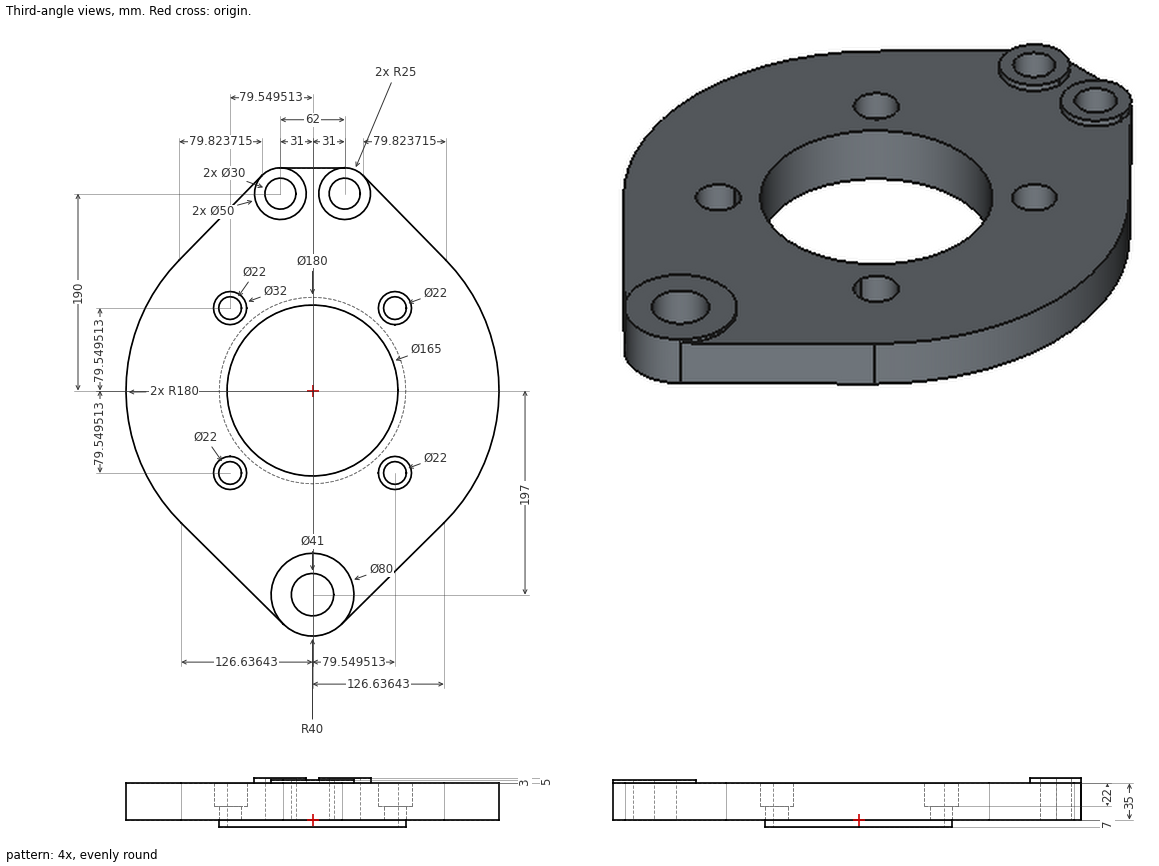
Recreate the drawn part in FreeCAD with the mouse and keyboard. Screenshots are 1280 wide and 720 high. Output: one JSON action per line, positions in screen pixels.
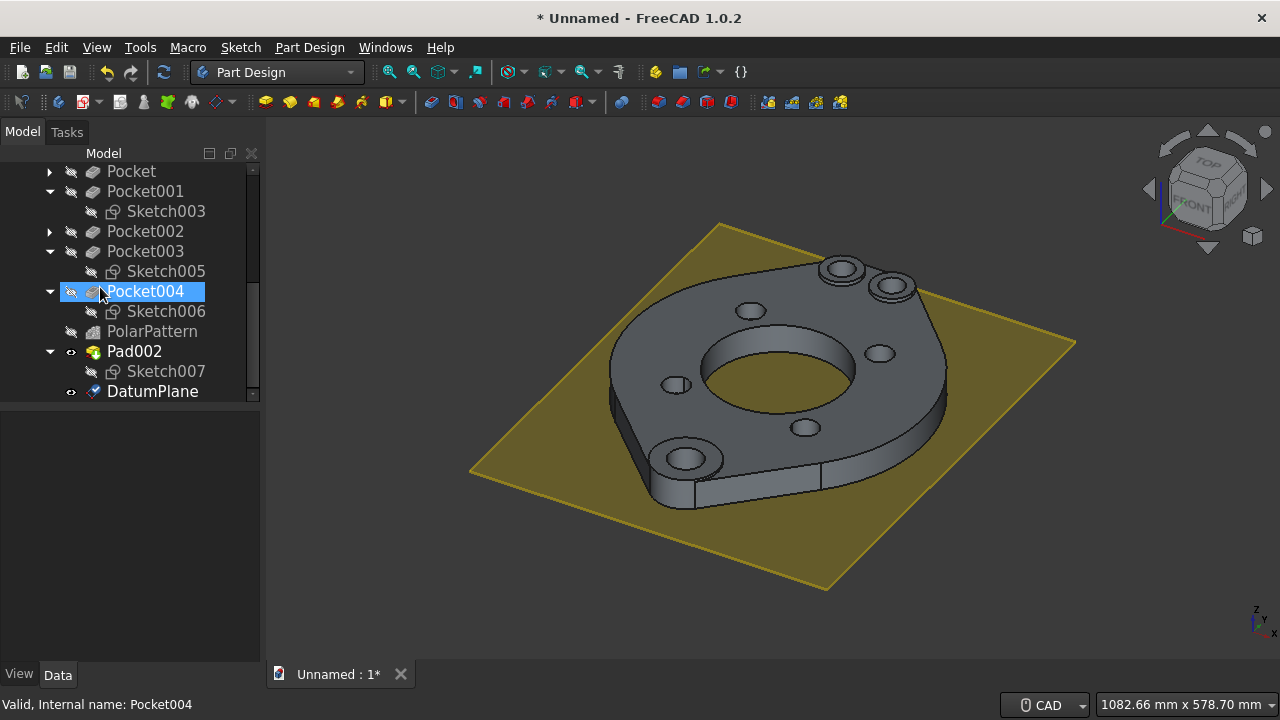
{"action": "left_click", "coordinate": [116, 392]}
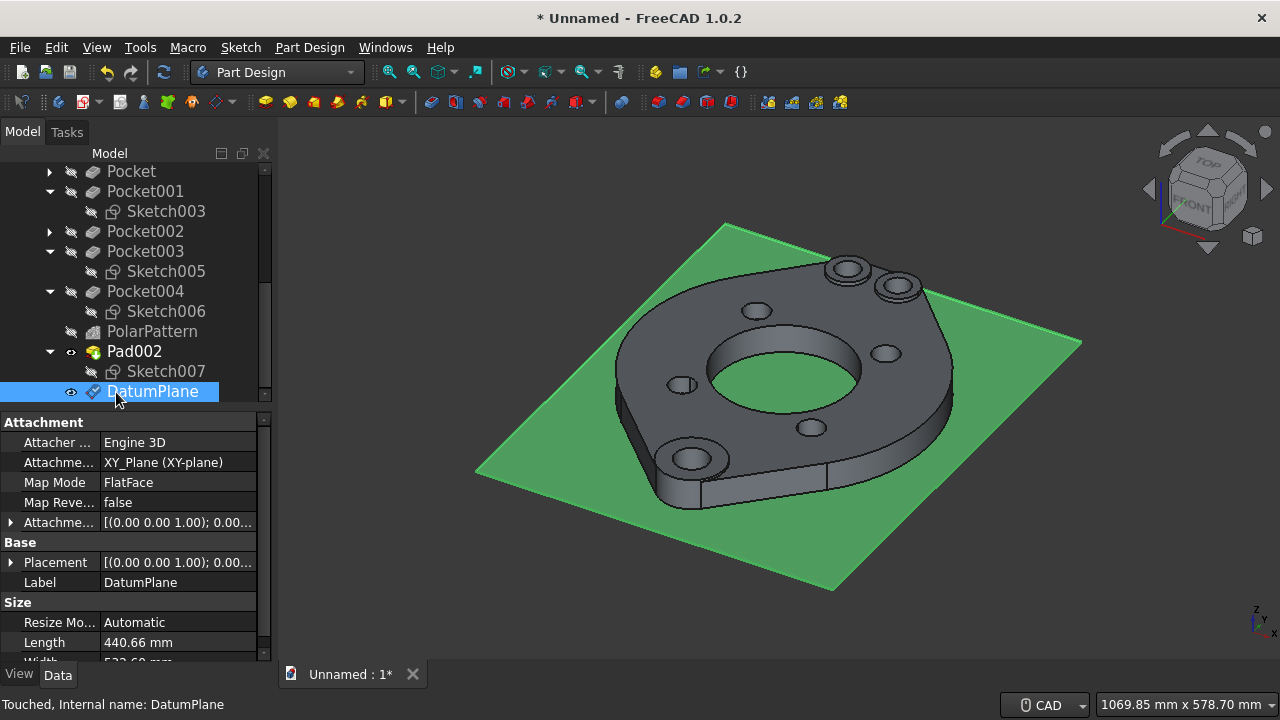
{"action": "left_click", "coordinate": [84, 102]}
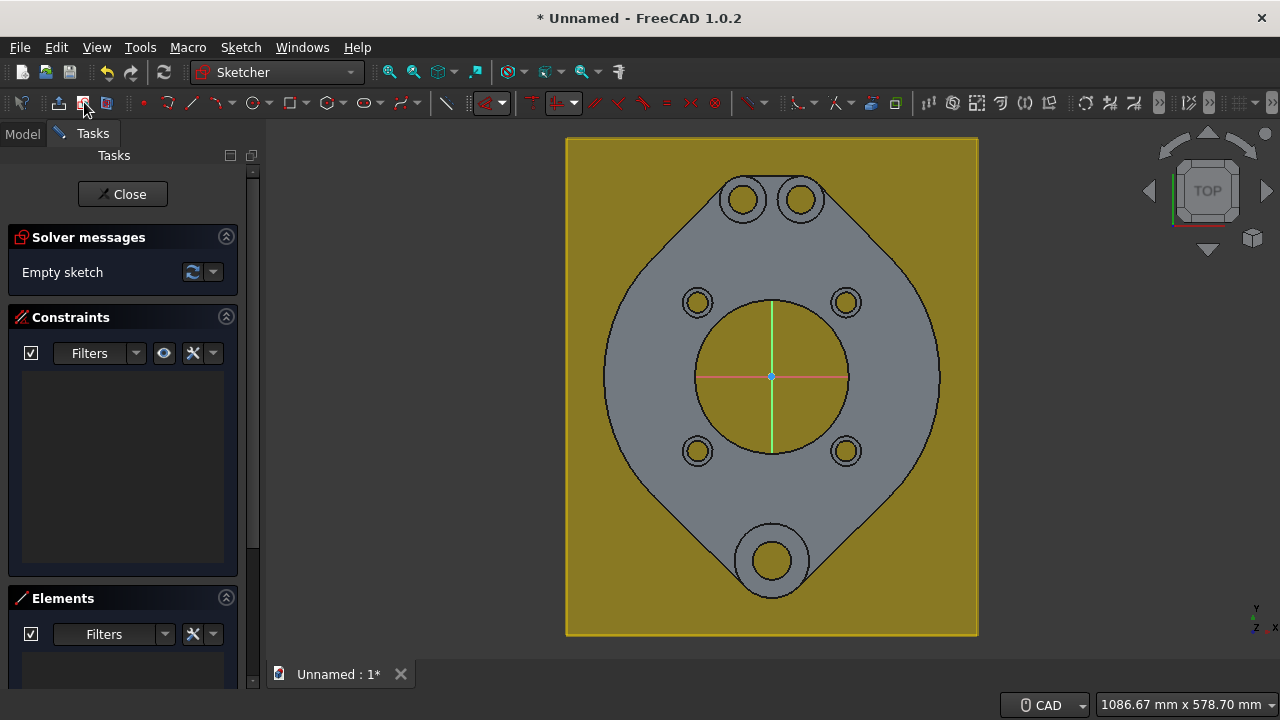
{"action": "left_click", "coordinate": [108, 104]}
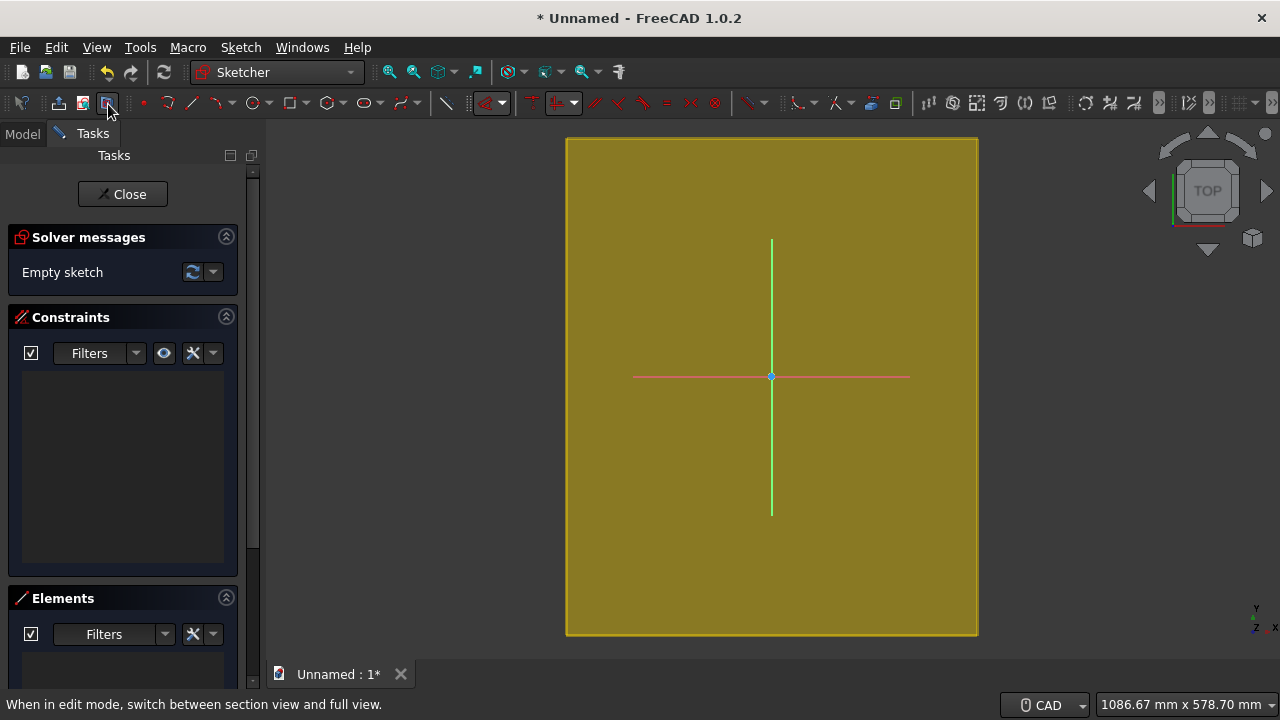
{"action": "scroll", "coordinate": [827, 367], "scroll_direction": "up", "scroll_amount": 4}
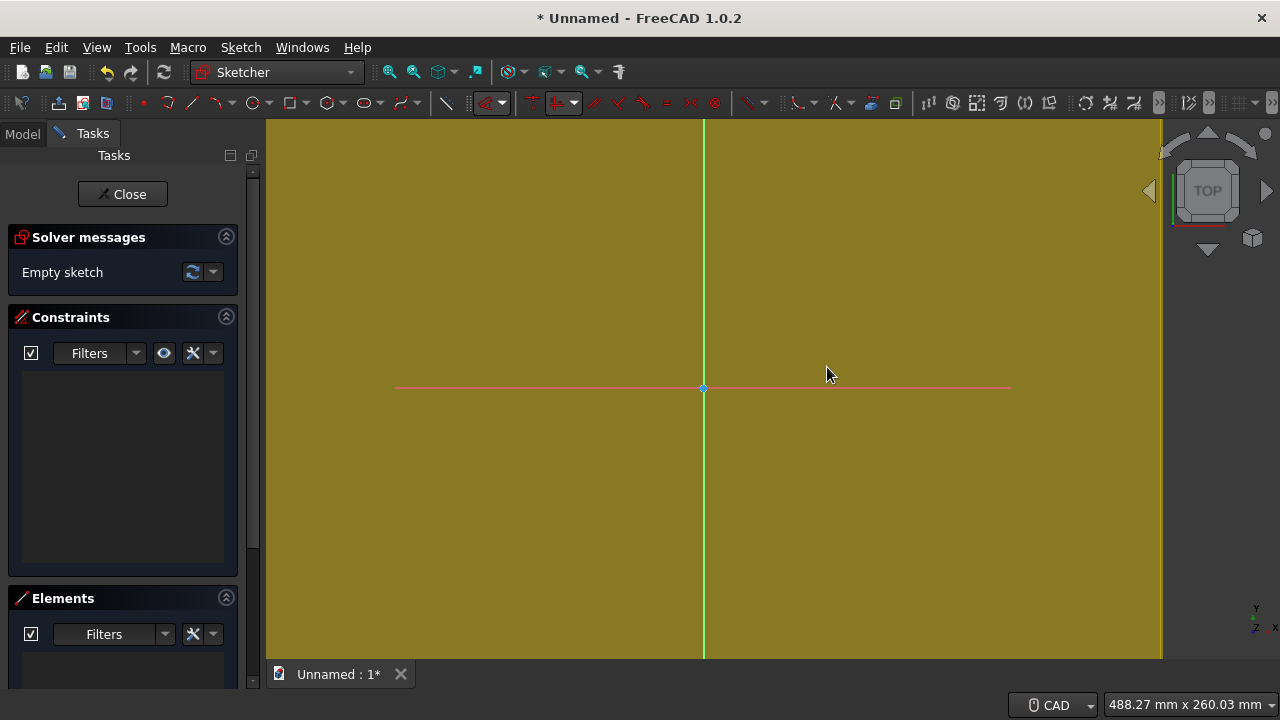
{"action": "key", "text": "g c"}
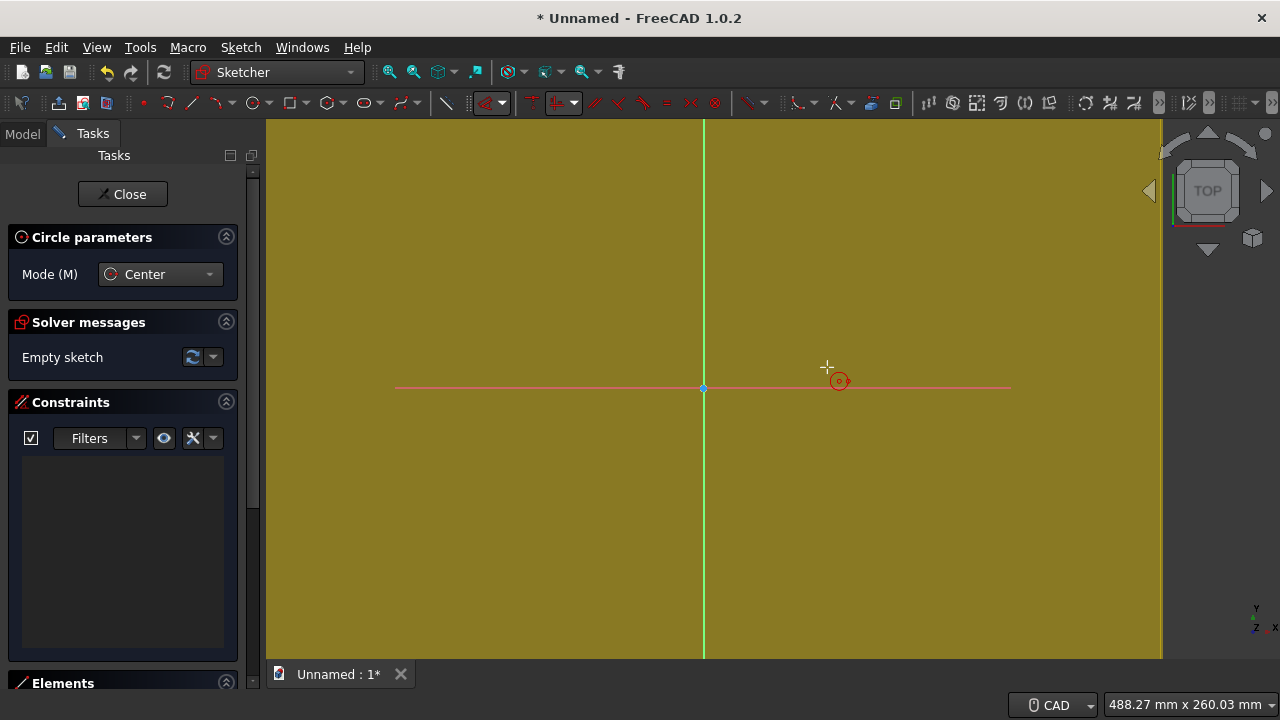
{"action": "left_click", "coordinate": [704, 388]}
{"action": "left_click", "coordinate": [836, 256]}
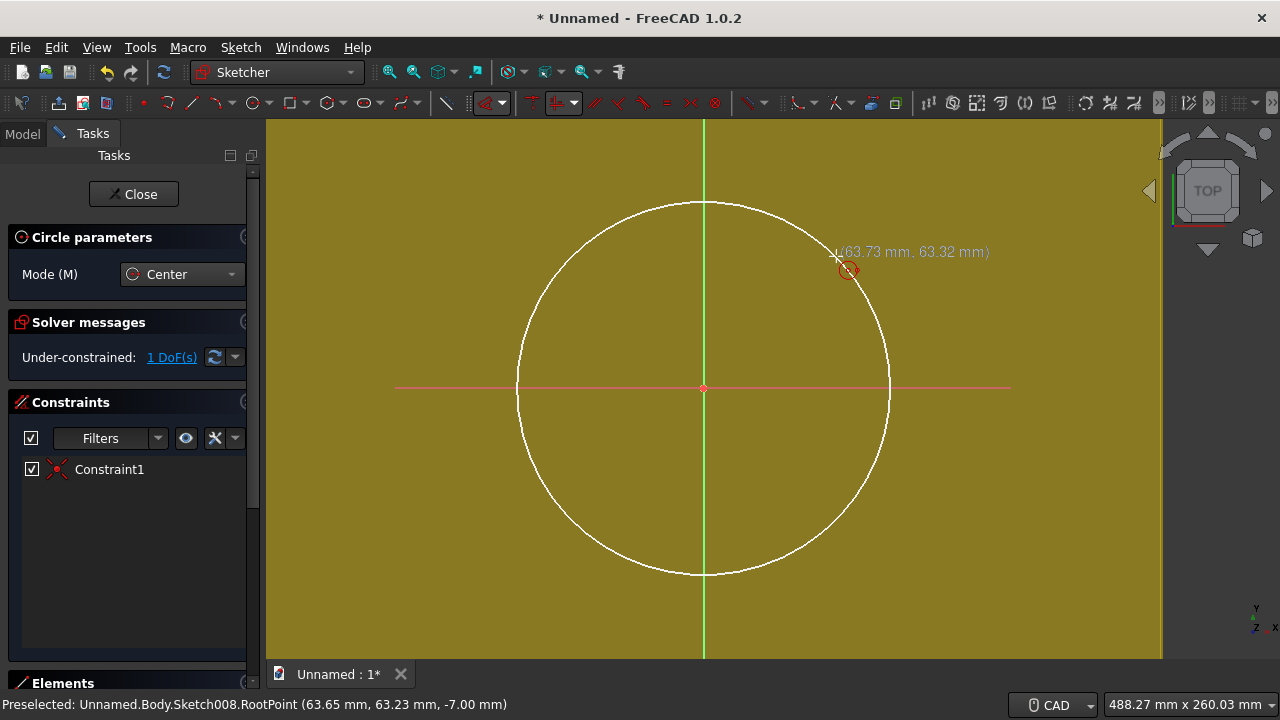
{"action": "left_click", "coordinate": [704, 388]}
{"action": "left_click", "coordinate": [825, 267]}
{"action": "key", "text": "Escape"}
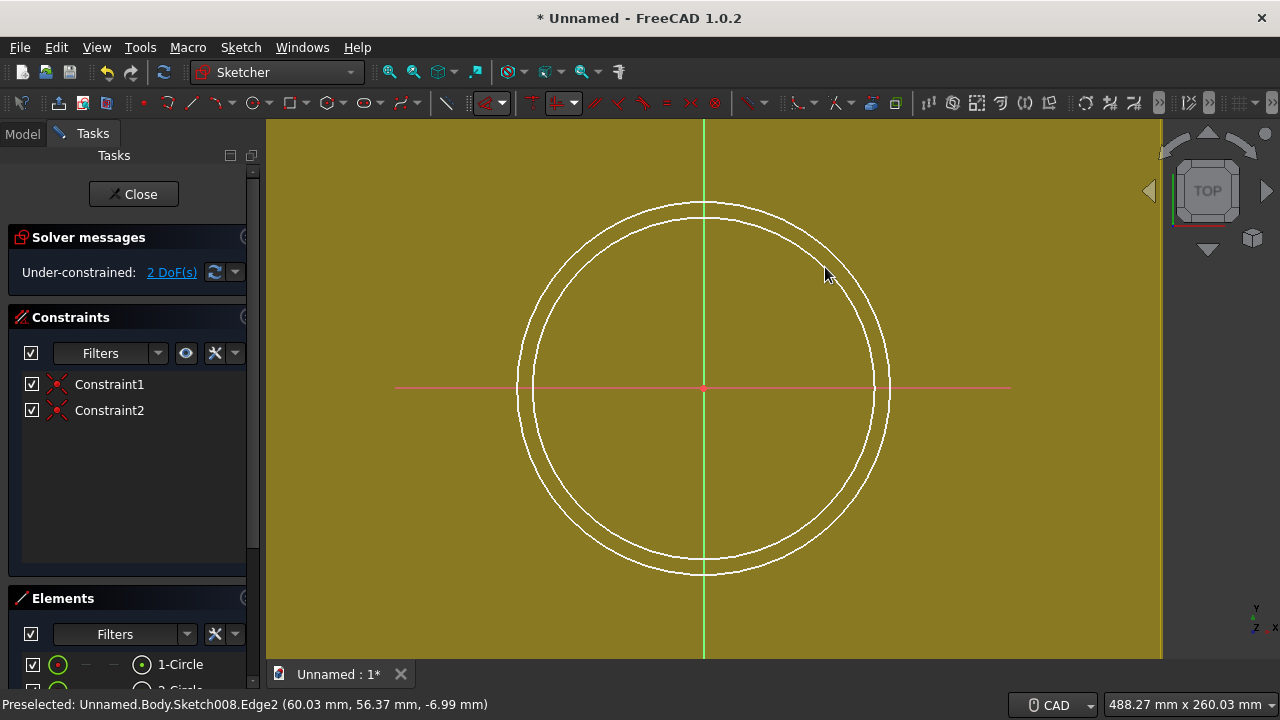
{"action": "left_click", "coordinate": [835, 256]}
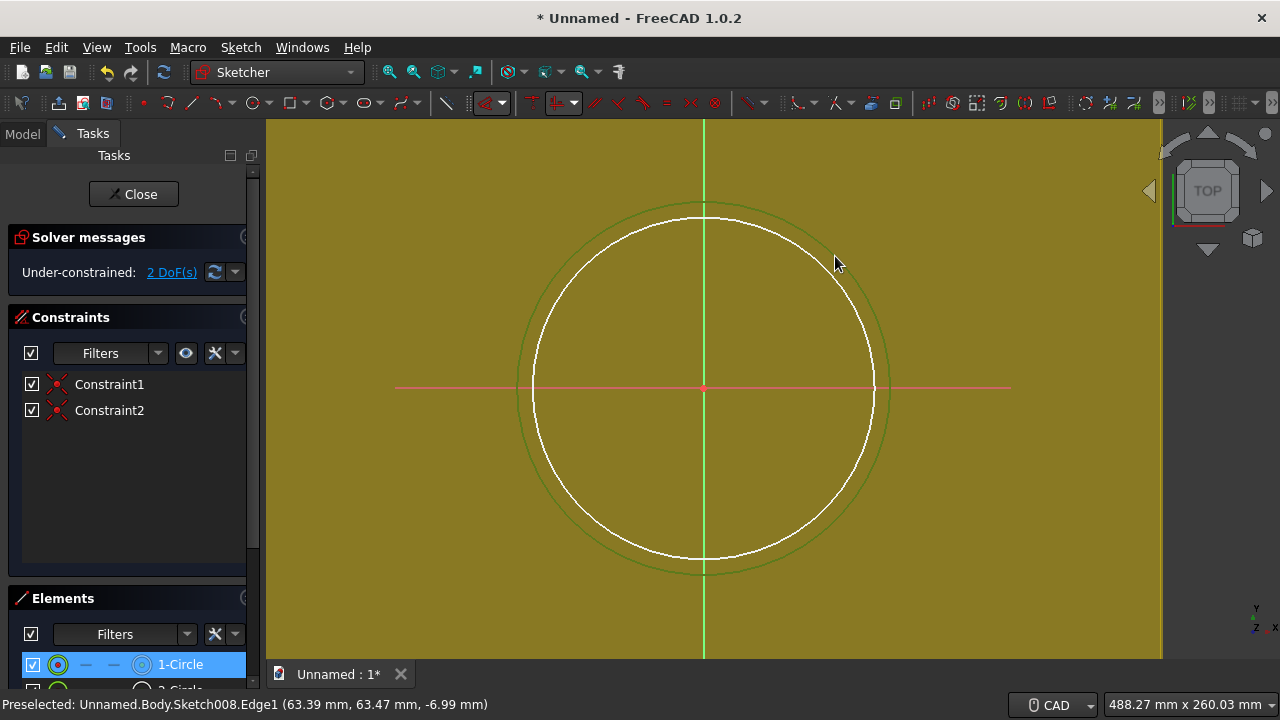
{"action": "key", "text": "k o"}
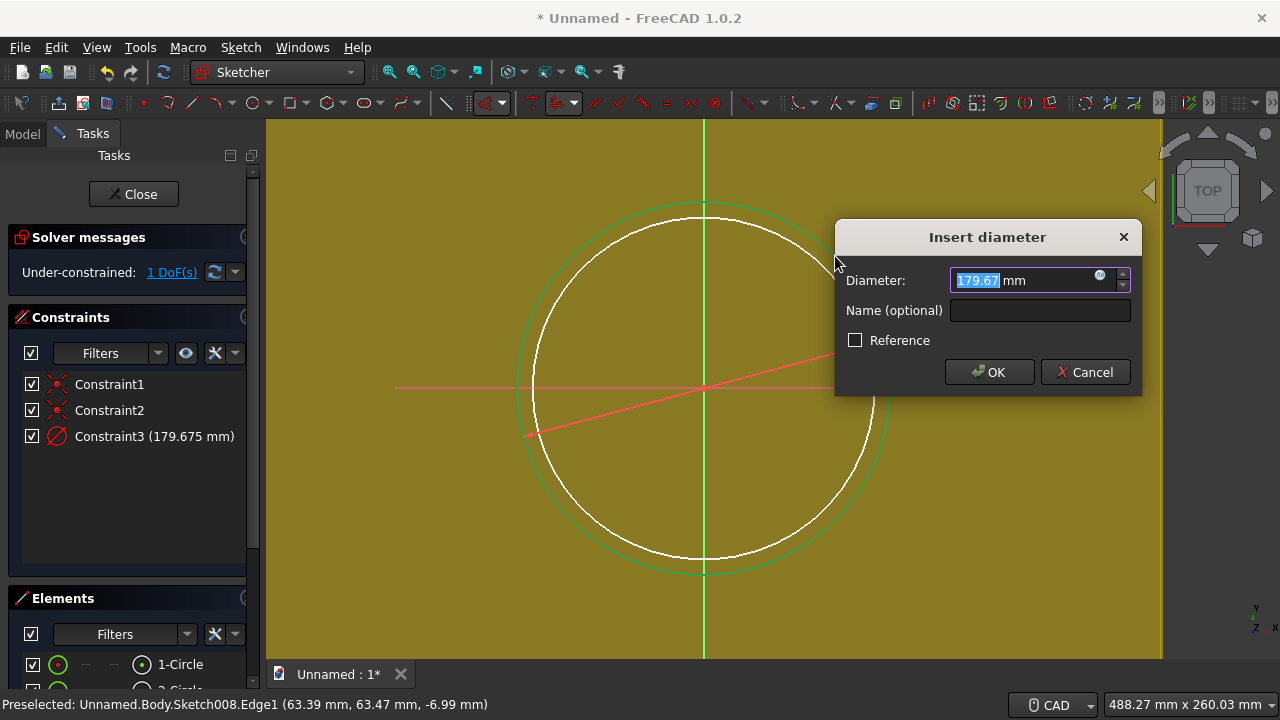
{"action": "type", "text": "180"}
{"action": "key", "text": "Return"}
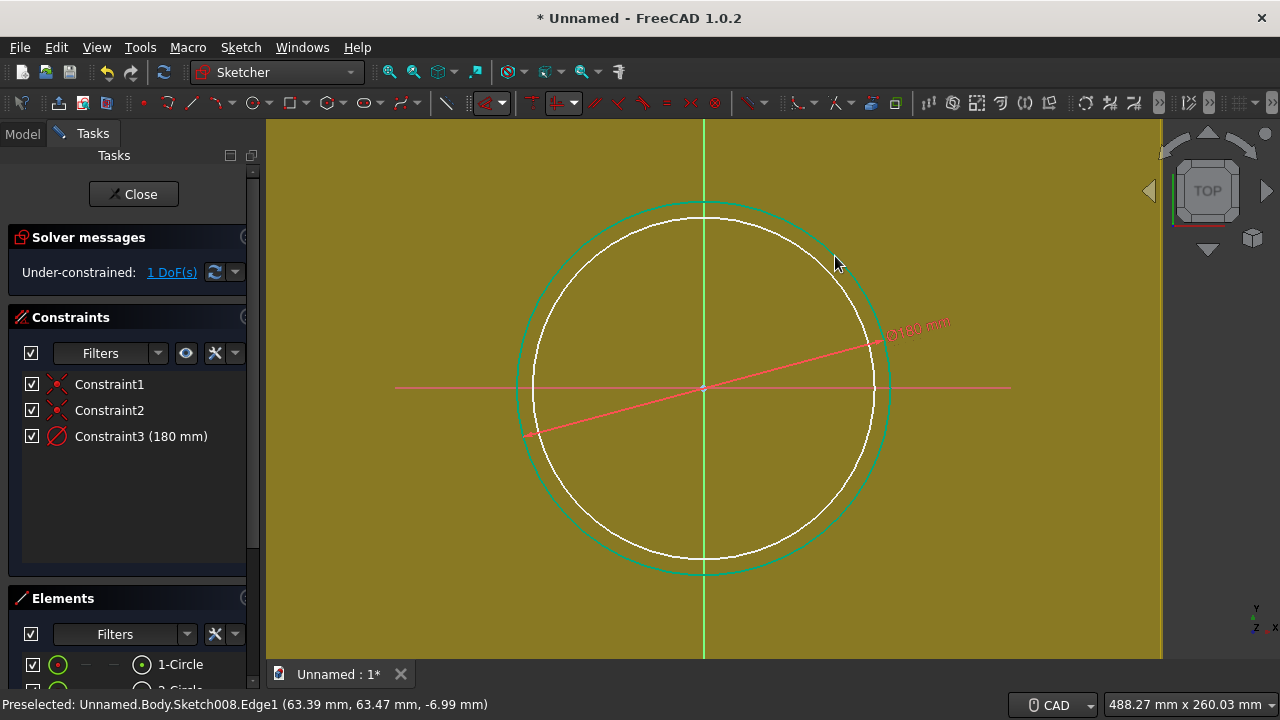
{"action": "left_click", "coordinate": [824, 267]}